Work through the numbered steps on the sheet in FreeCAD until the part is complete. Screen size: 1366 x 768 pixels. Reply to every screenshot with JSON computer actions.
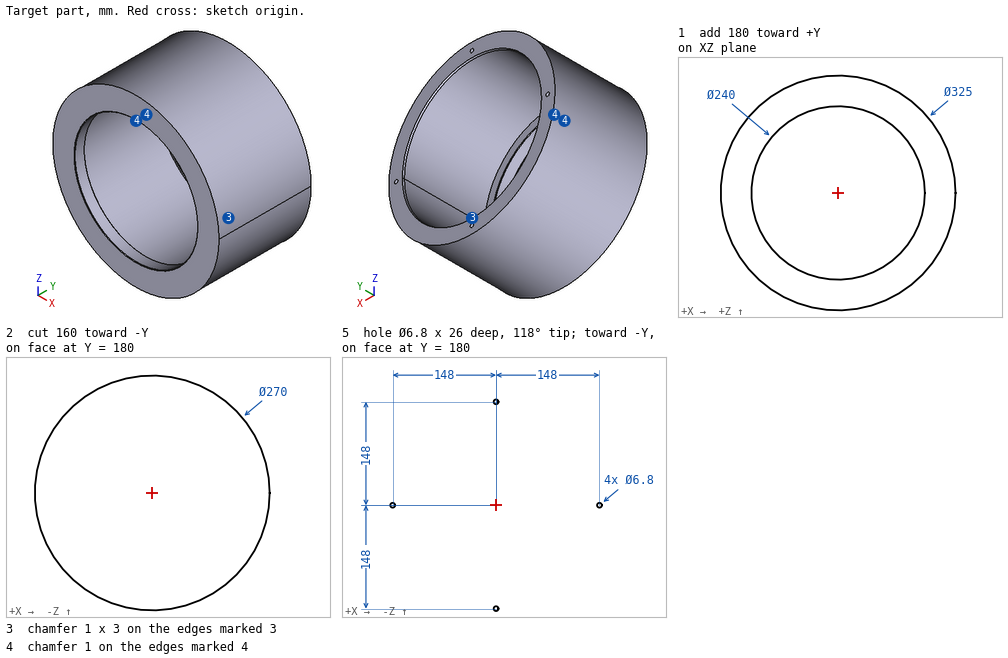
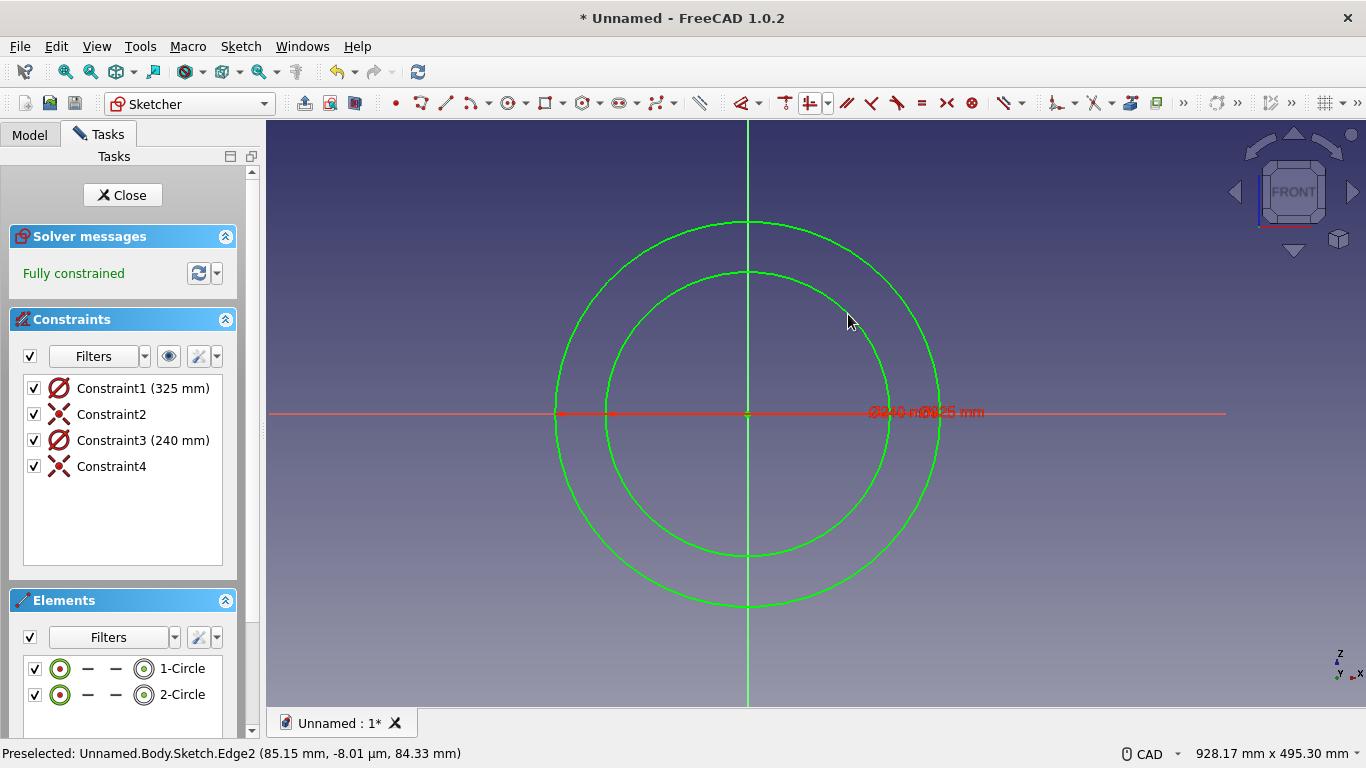
{"action": "left_click", "coordinate": [123, 195]}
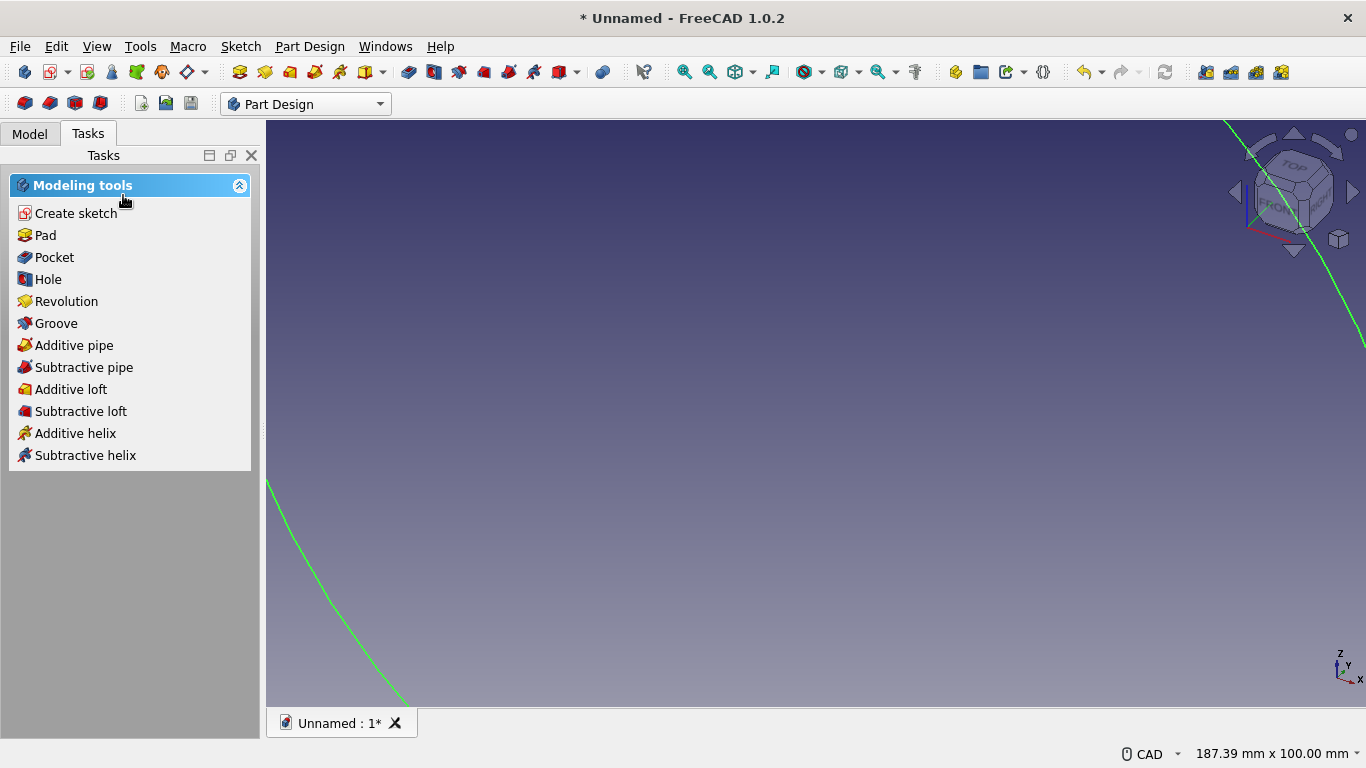
{"action": "left_click", "coordinate": [240, 72]}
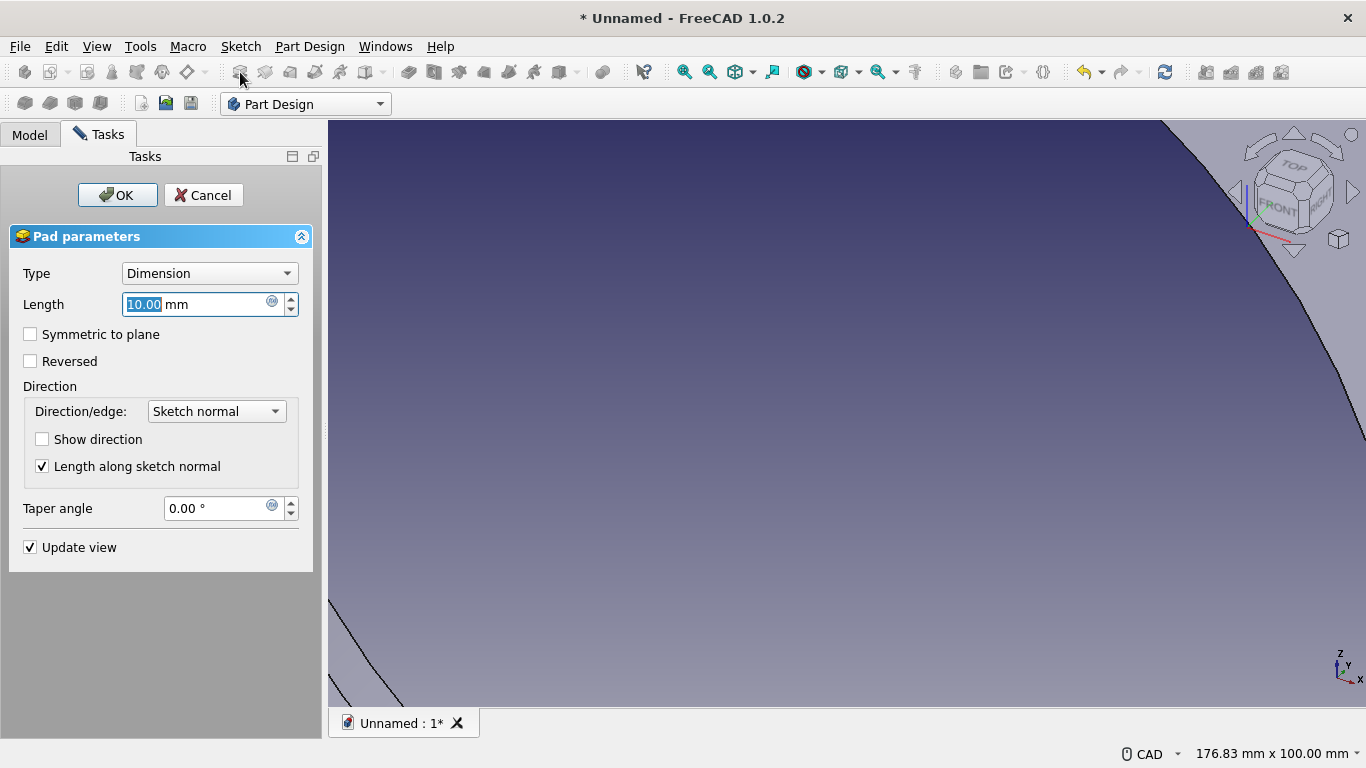
{"action": "type", "text": "180"}
{"action": "key", "text": "Tab"}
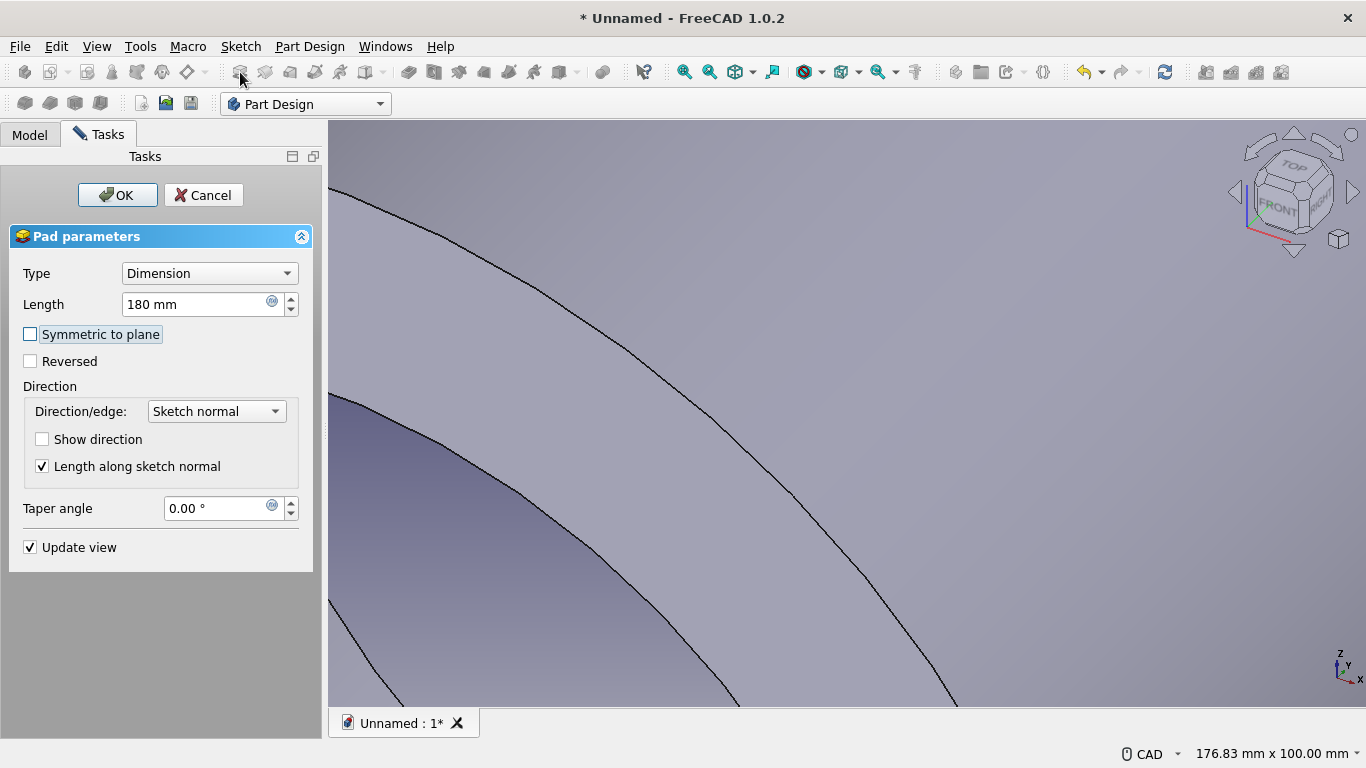
{"action": "left_click", "coordinate": [31, 361]}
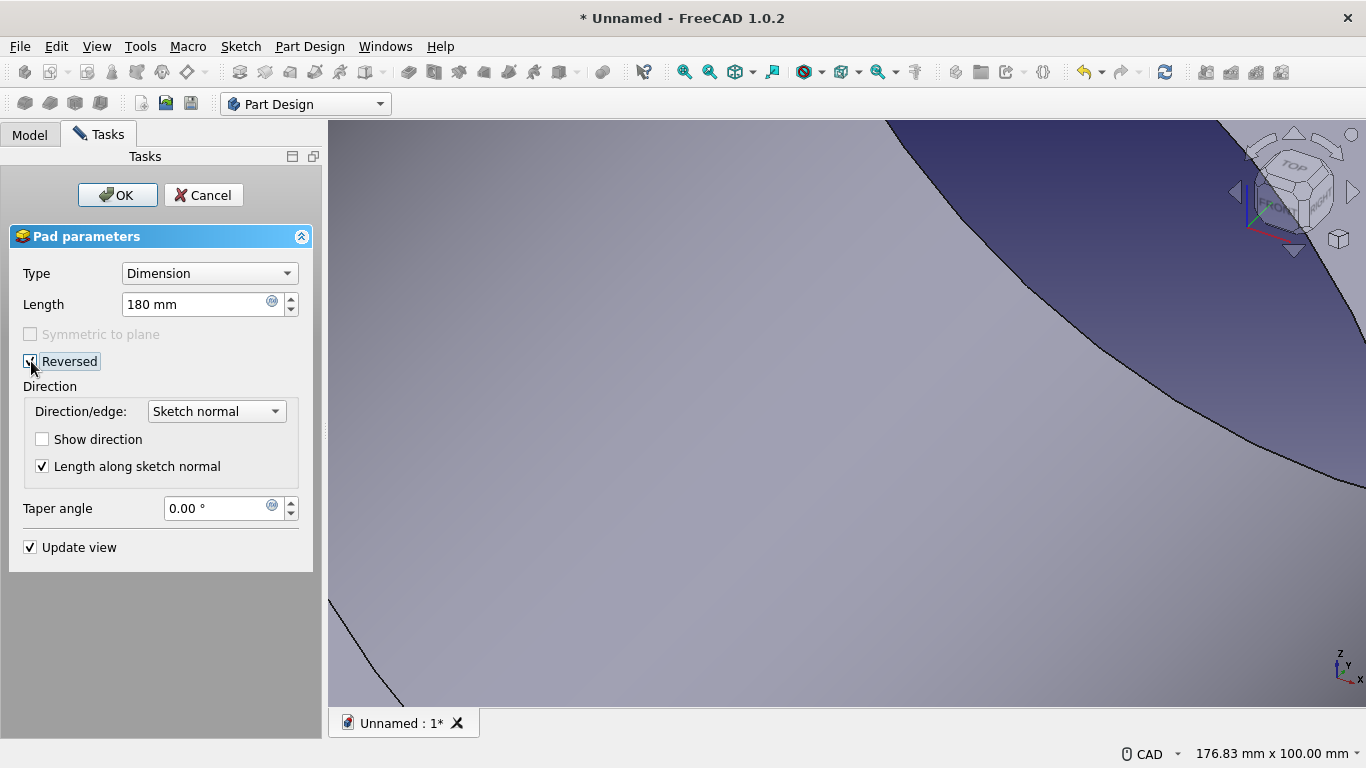
{"action": "left_click", "coordinate": [118, 195]}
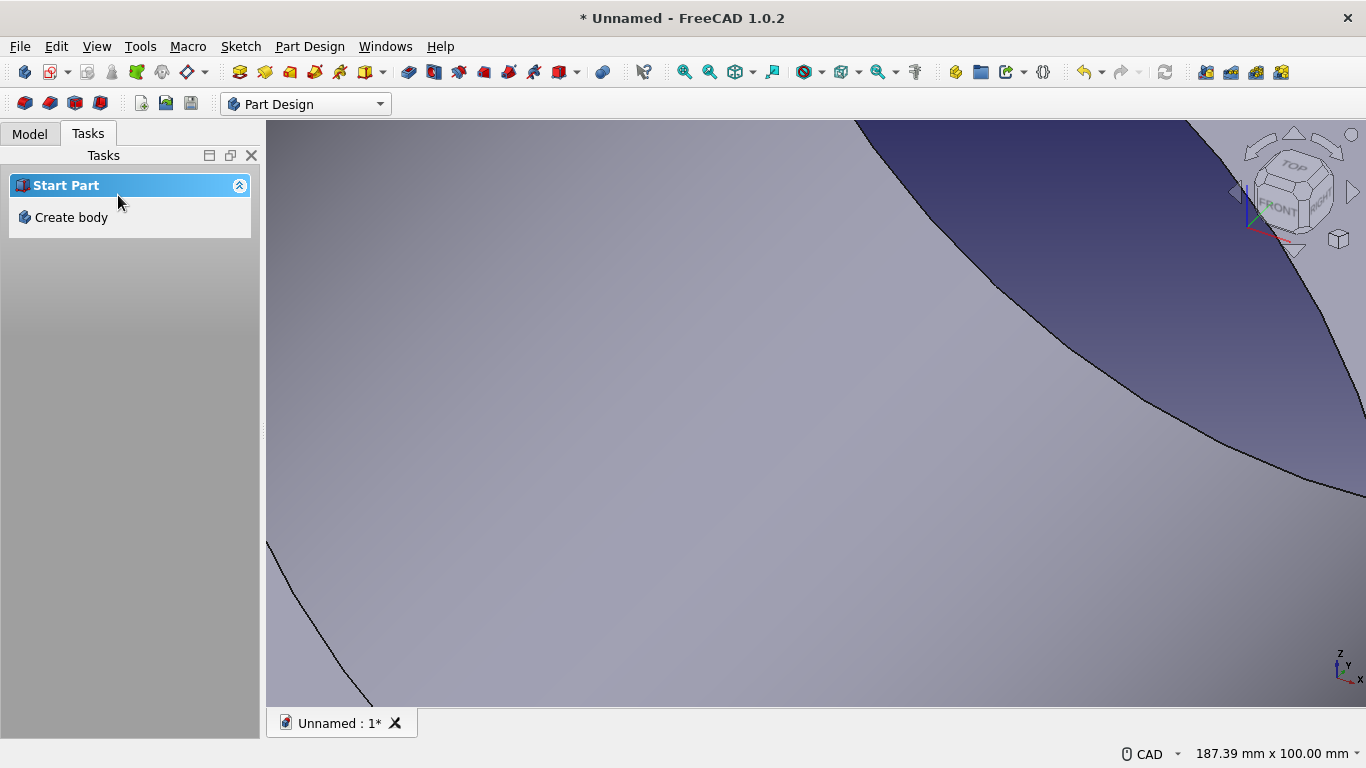
{"action": "left_click", "coordinate": [685, 72]}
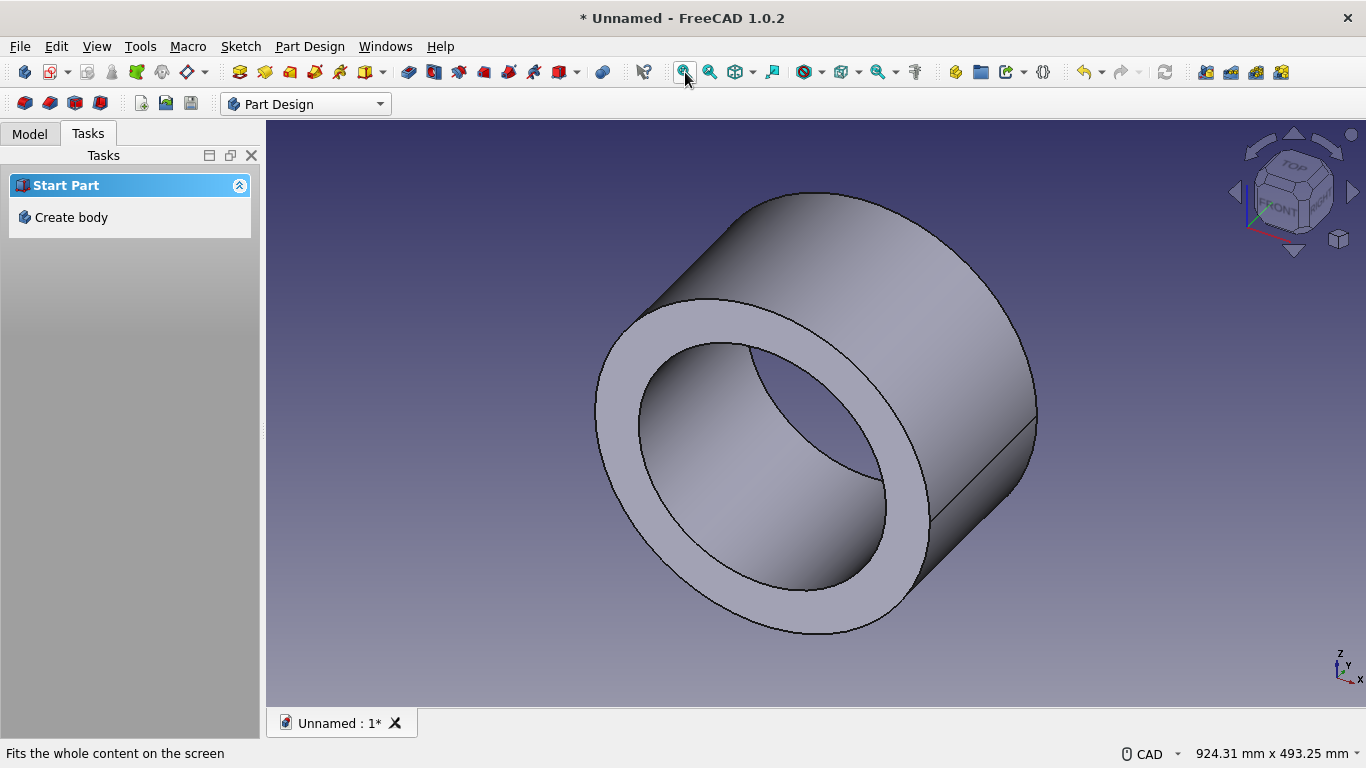
{"action": "key", "text": "4"}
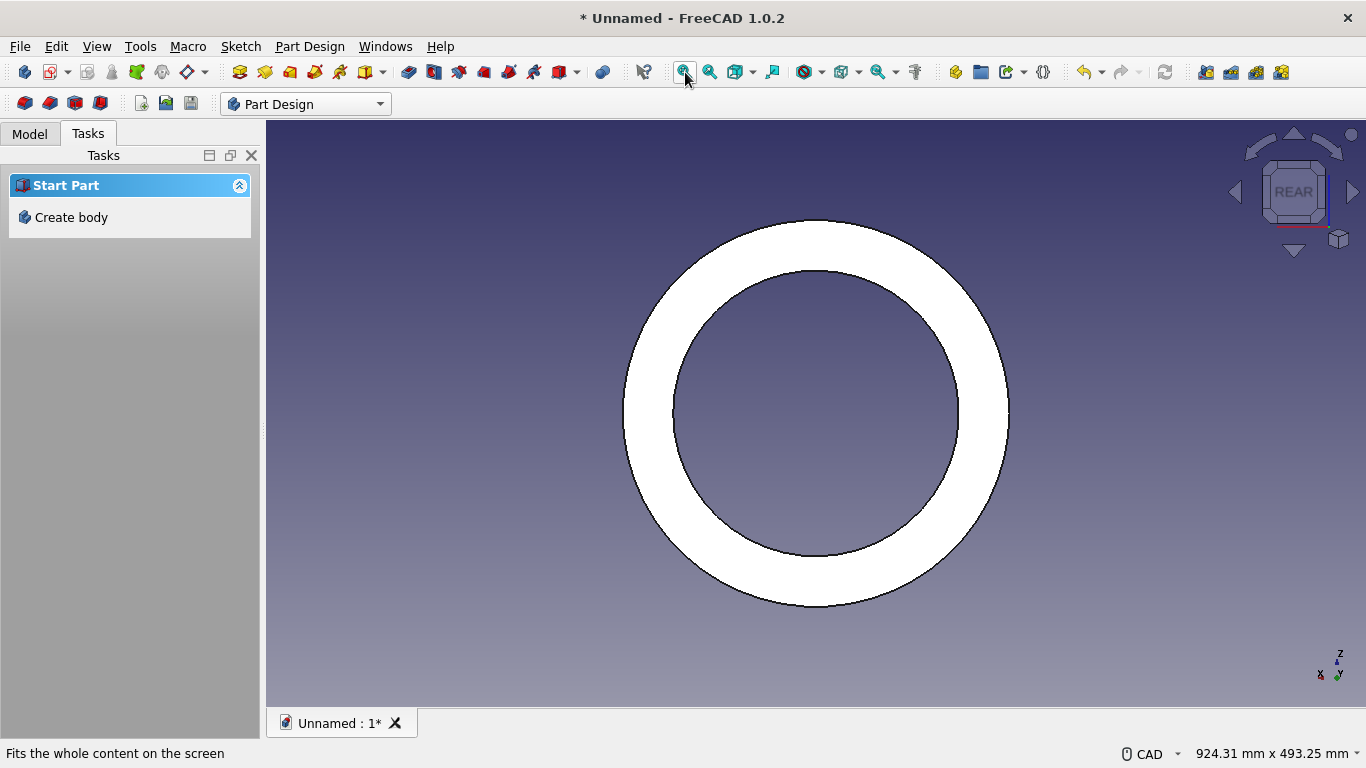
{"action": "left_click", "coordinate": [816, 247]}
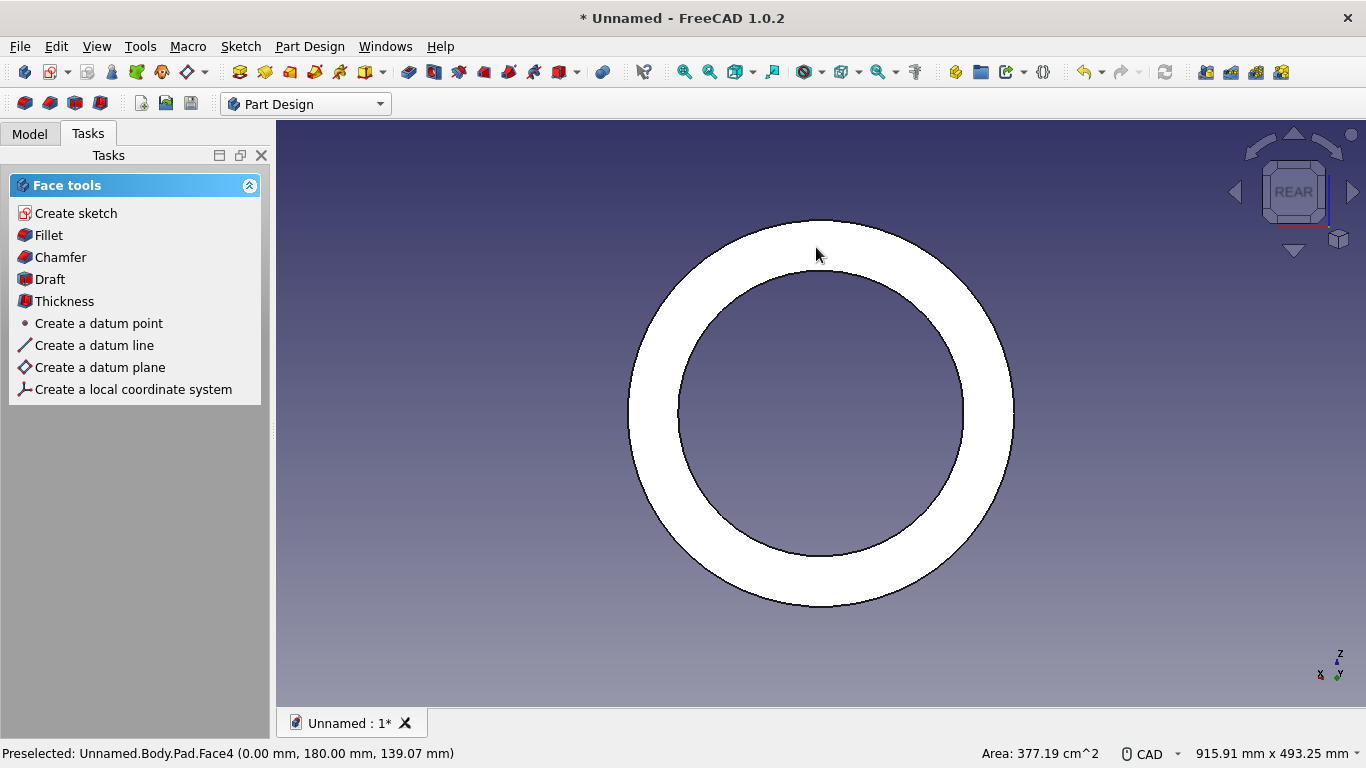
{"action": "left_click", "coordinate": [50, 72]}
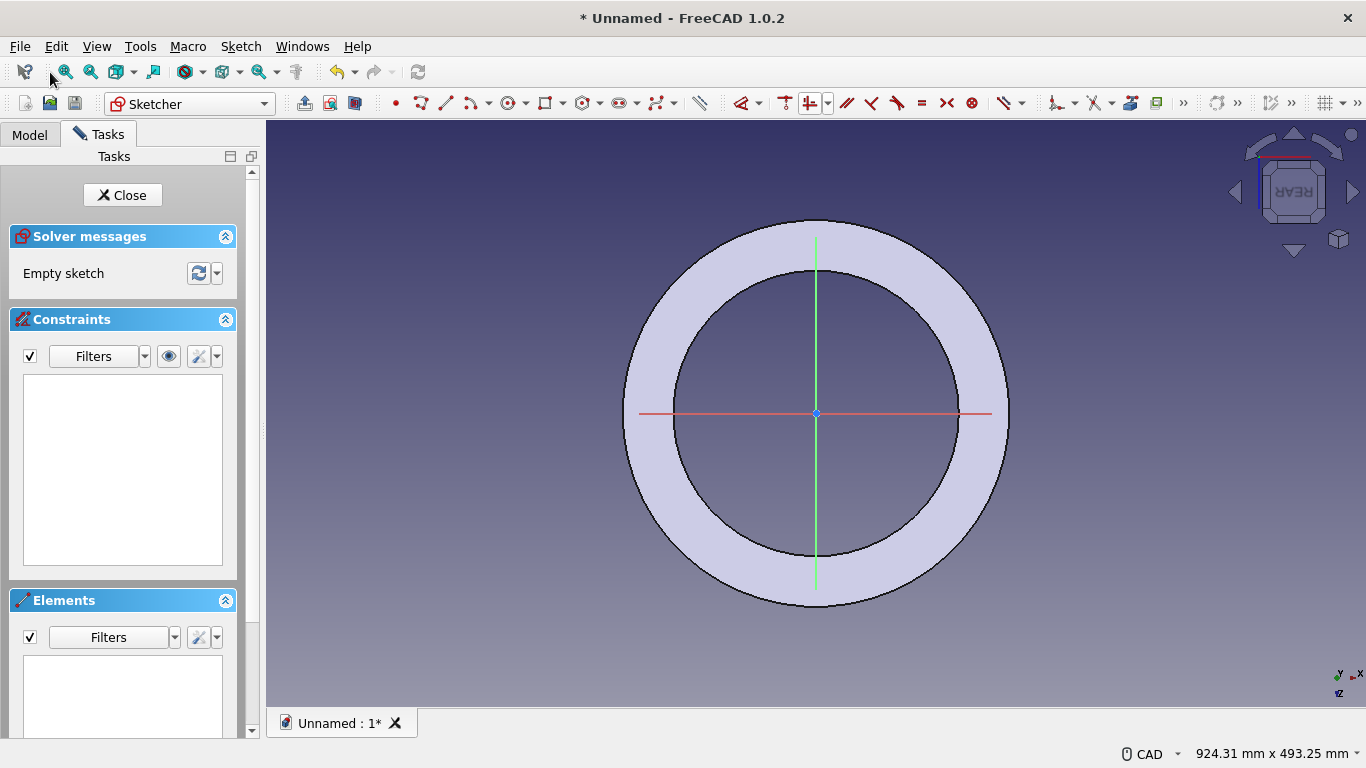
{"action": "left_click", "coordinate": [508, 104]}